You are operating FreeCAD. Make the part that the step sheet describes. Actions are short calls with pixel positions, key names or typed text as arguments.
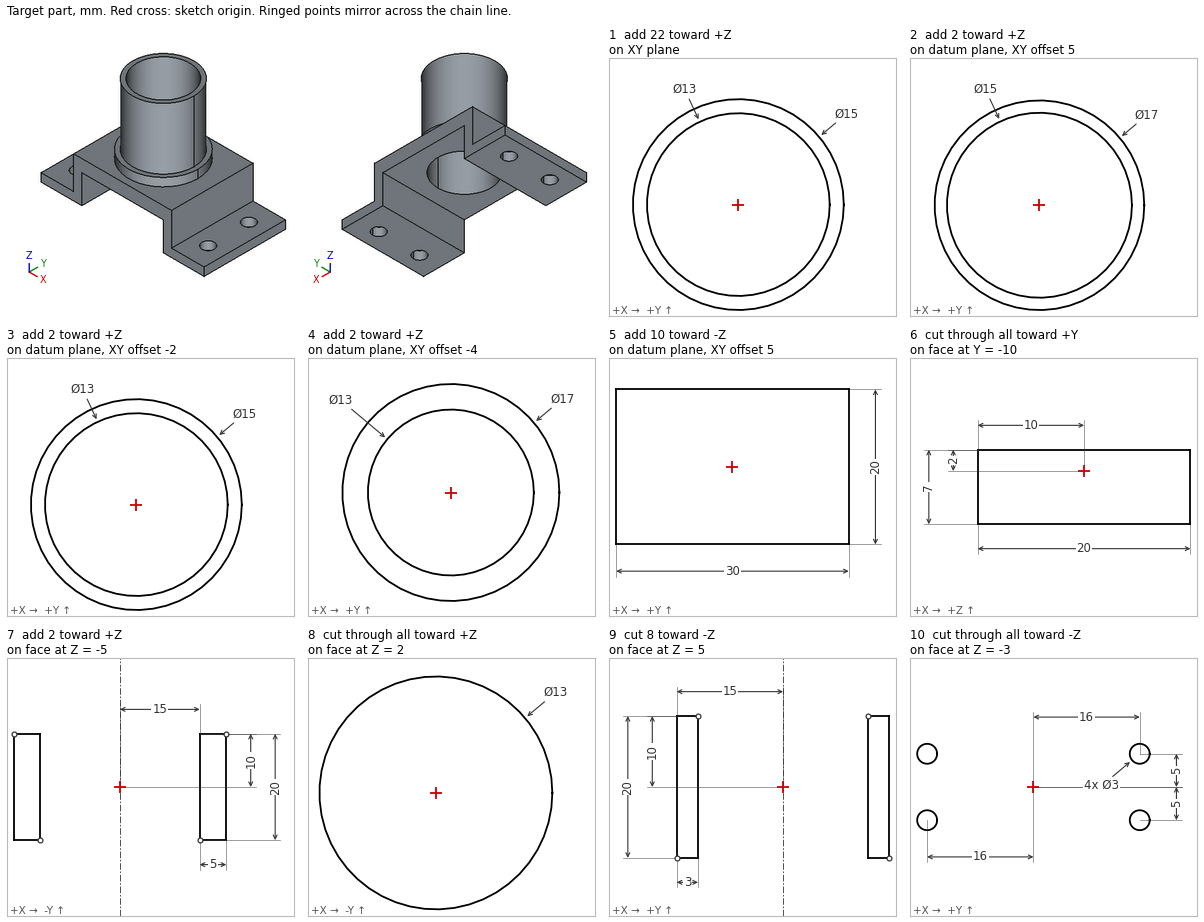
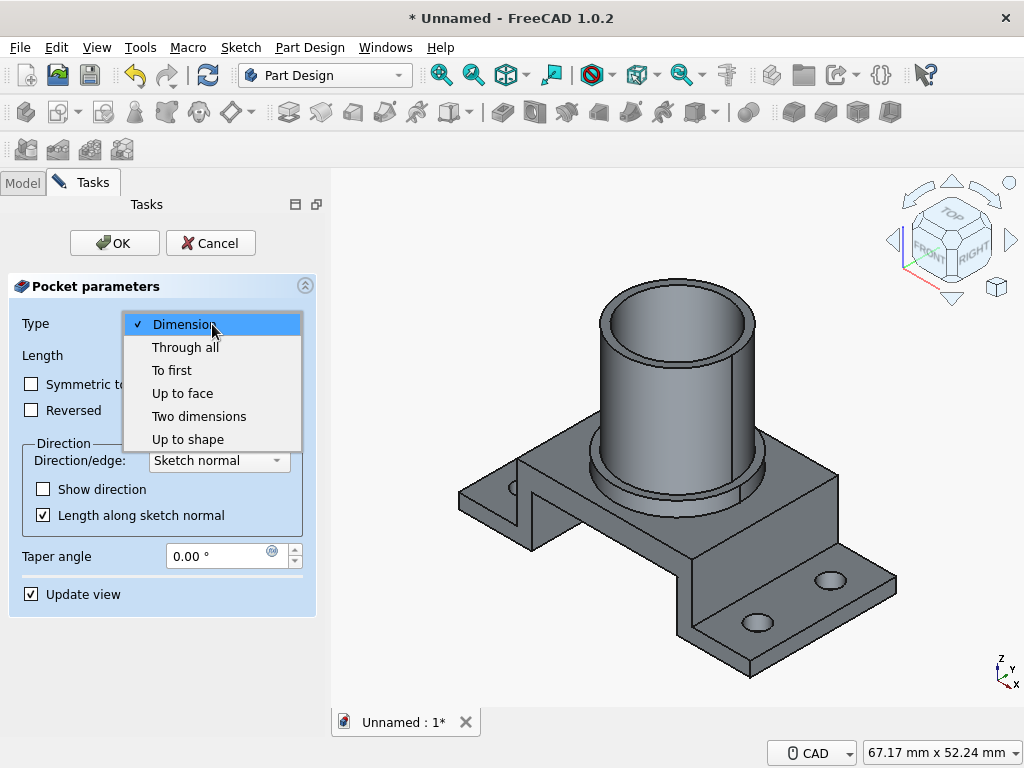
click(212, 348)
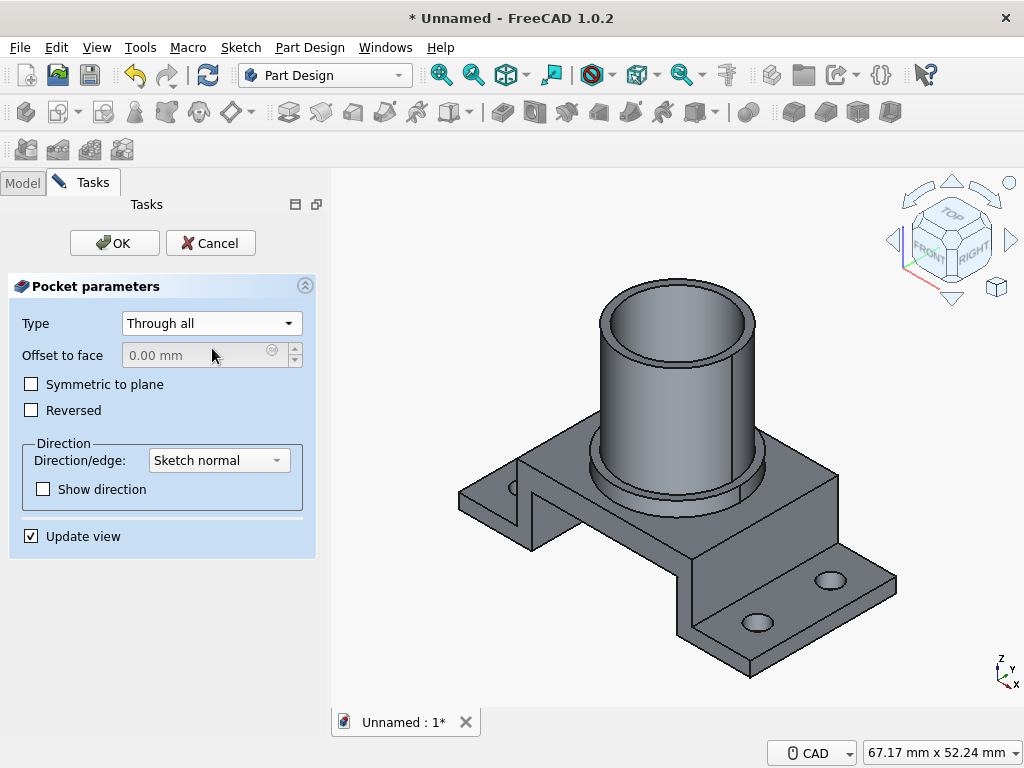
click(115, 243)